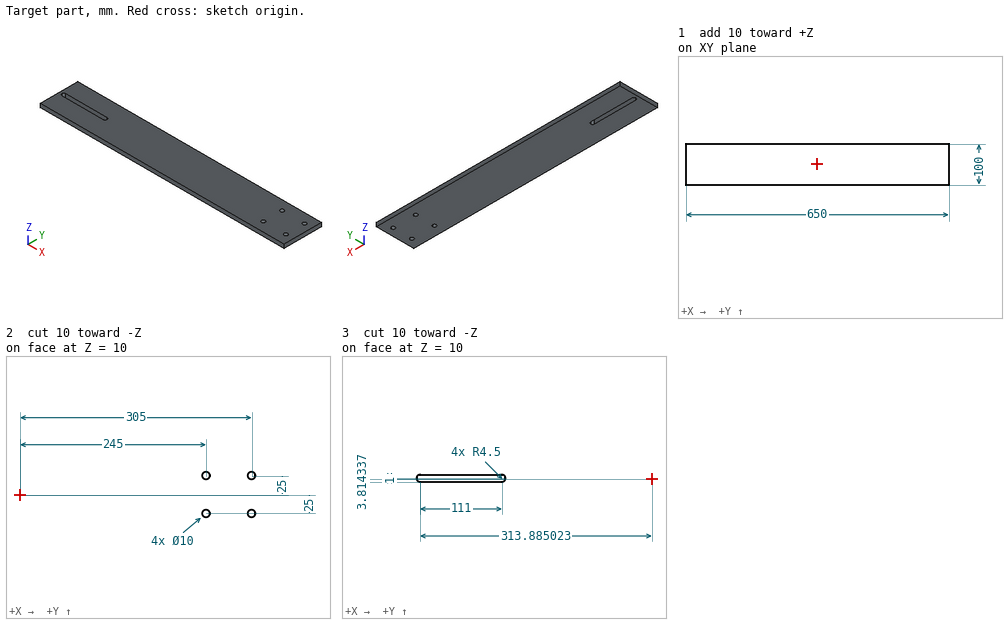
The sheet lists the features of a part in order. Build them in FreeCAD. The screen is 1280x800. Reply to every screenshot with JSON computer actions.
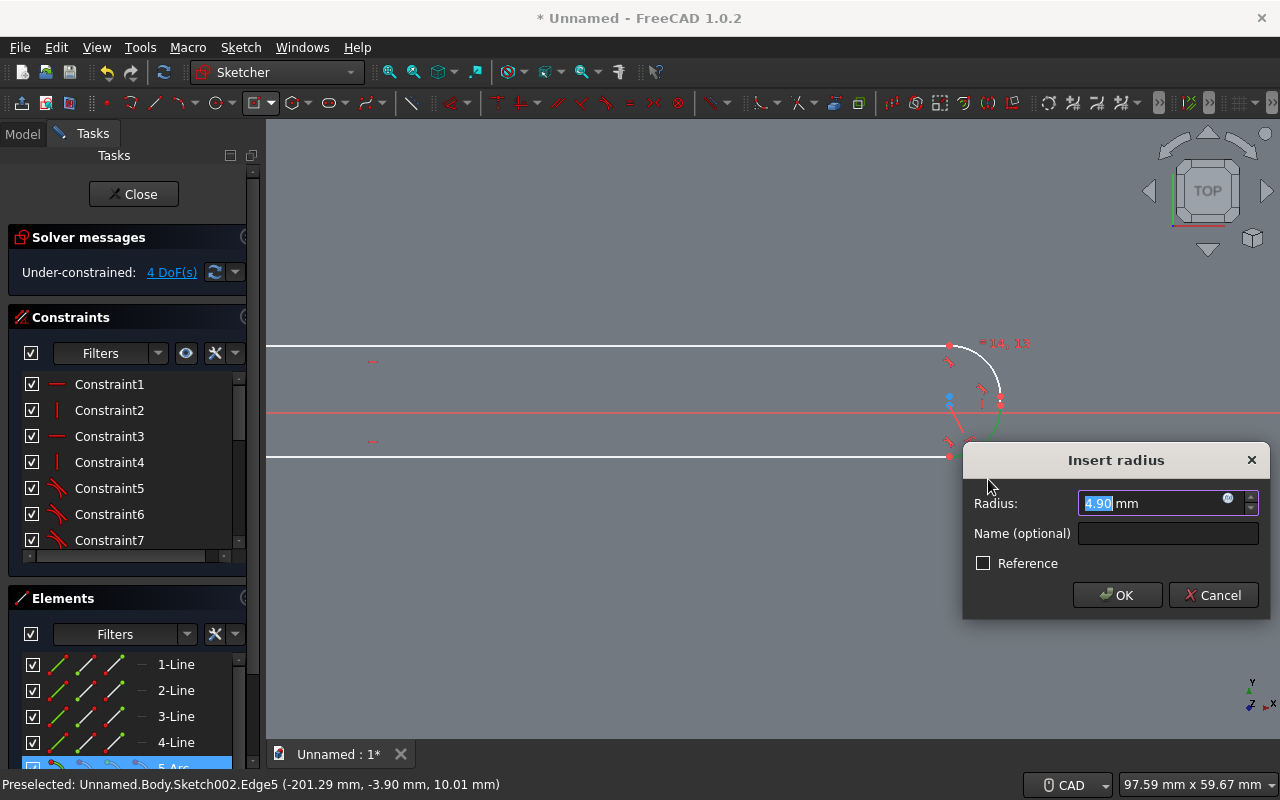
{"action": "type", "text": "4.5"}
{"action": "key", "text": "Return"}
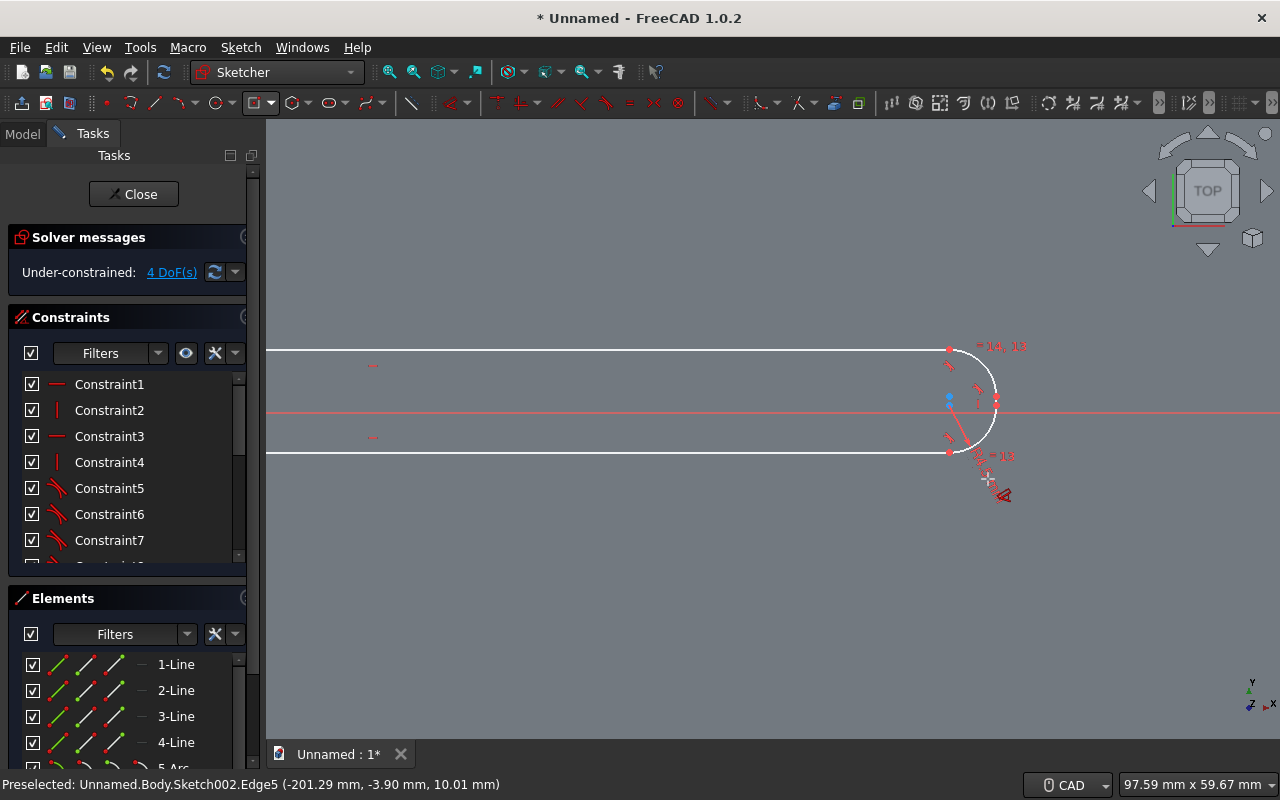
{"action": "scroll", "coordinate": [996, 401], "scroll_direction": "up", "scroll_amount": 7}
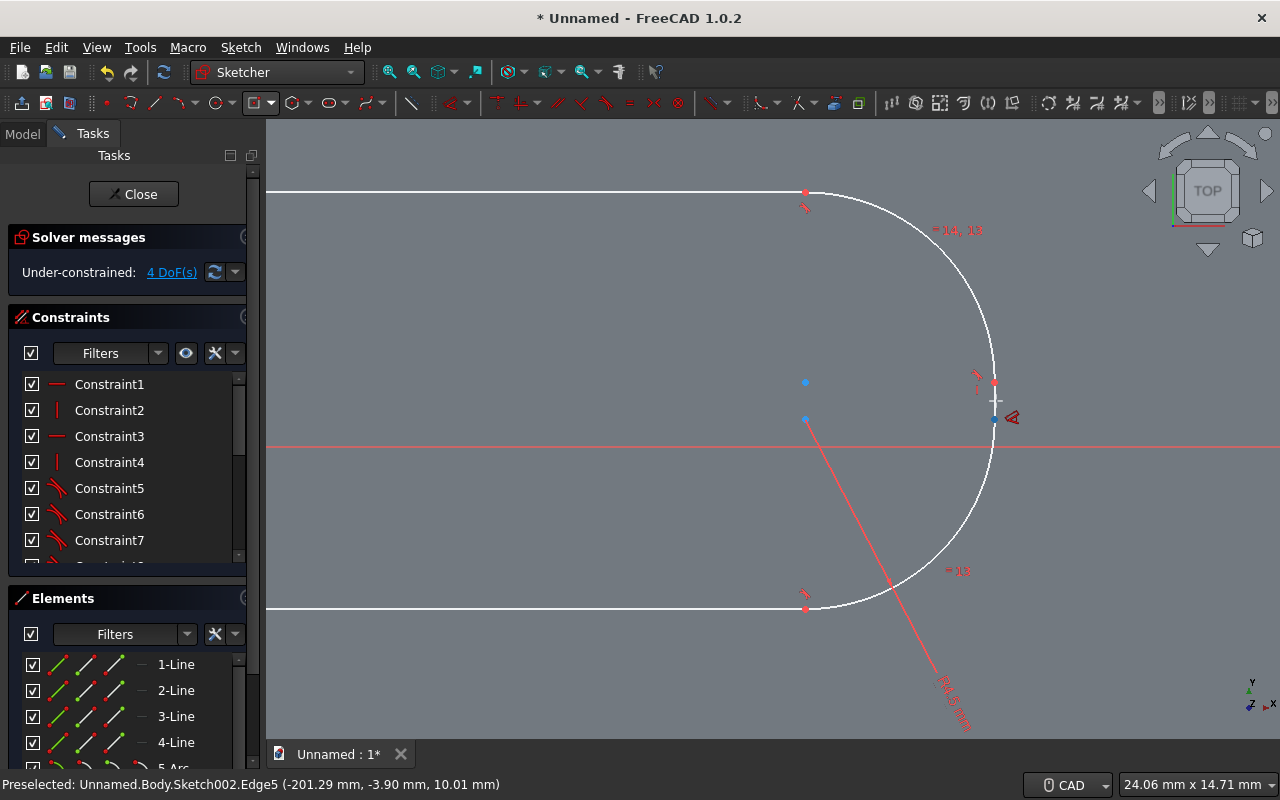
{"action": "left_click", "coordinate": [995, 401]}
{"action": "left_click", "coordinate": [1029, 401]}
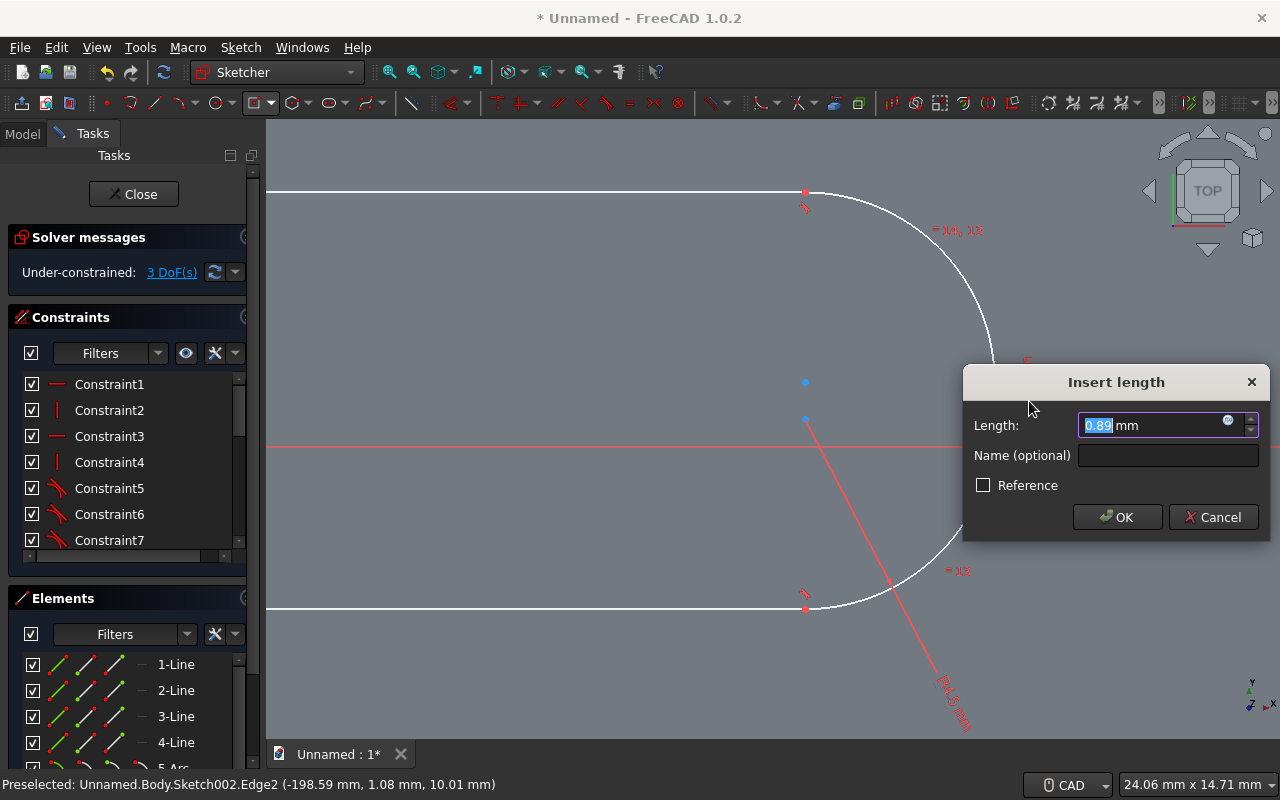
{"action": "type", "text": "1"}
{"action": "key", "text": "Return"}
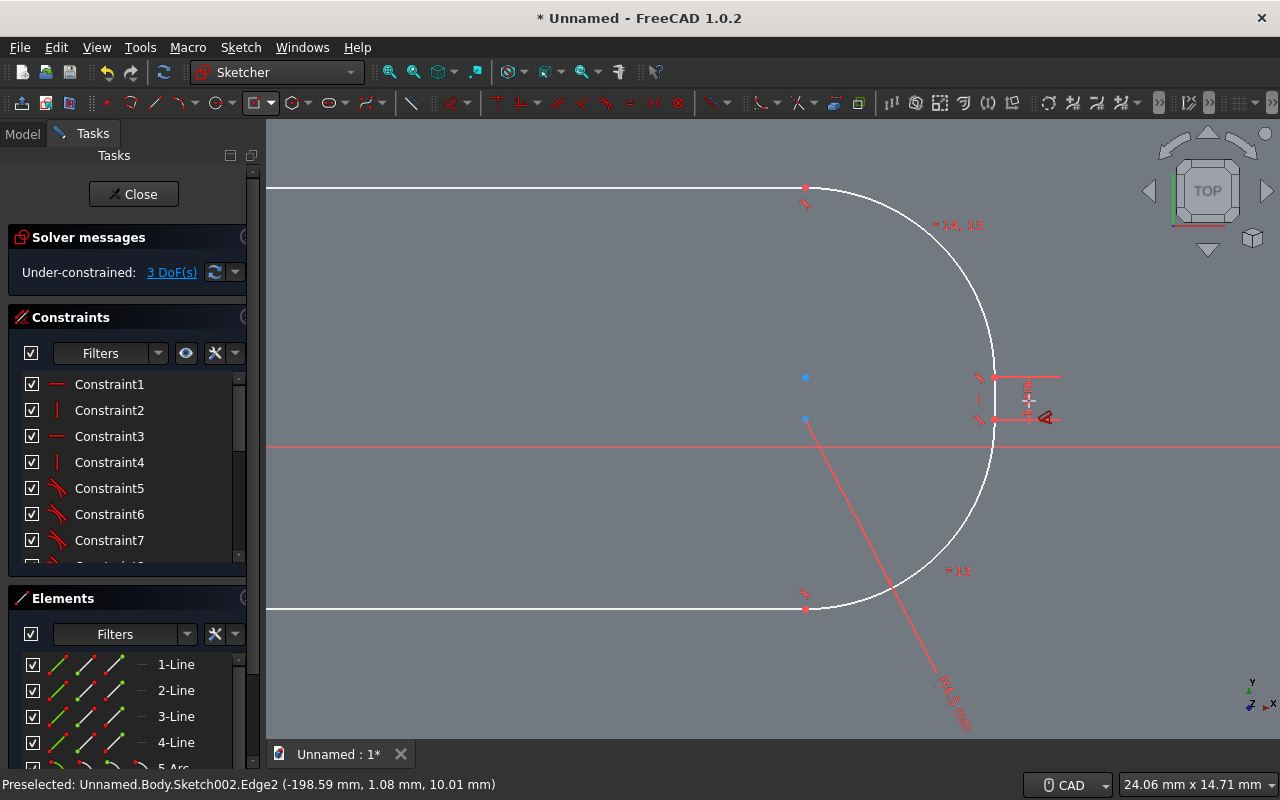
{"action": "scroll", "coordinate": [982, 433], "scroll_direction": "down", "scroll_amount": 11}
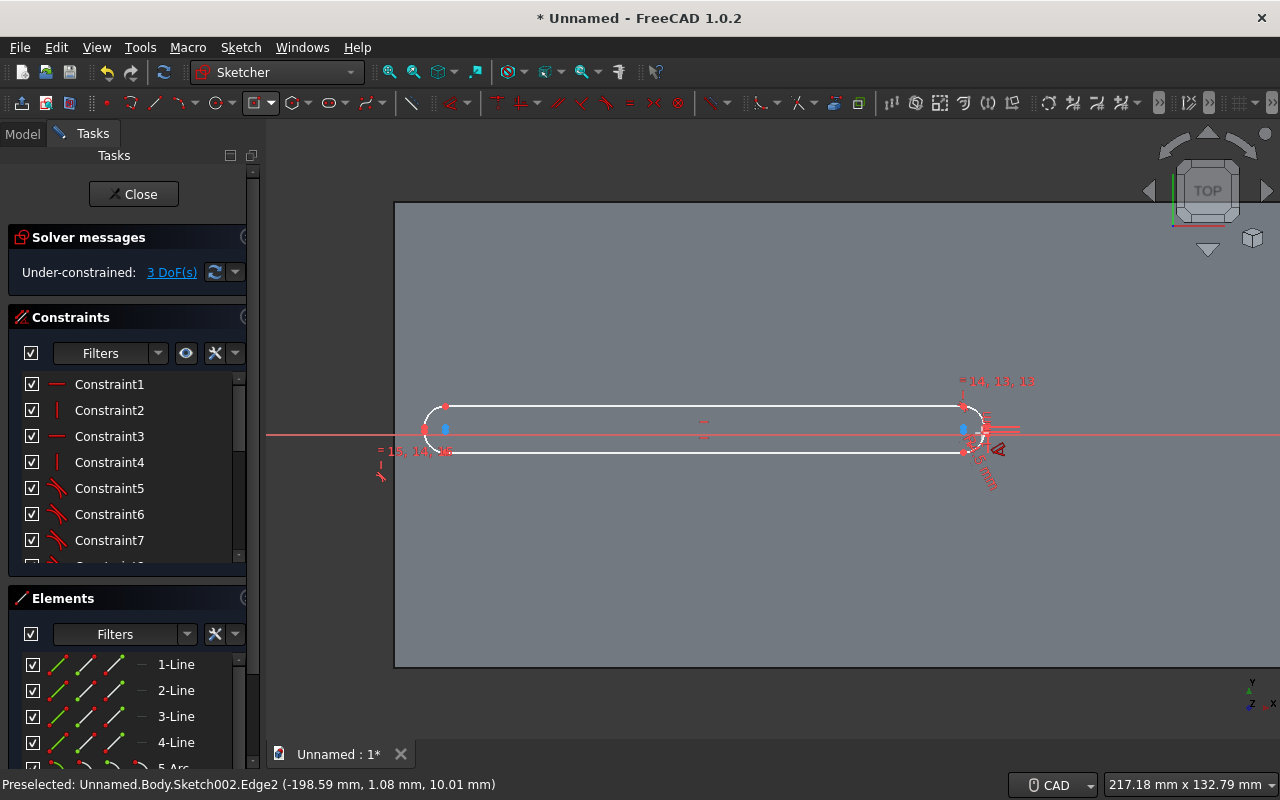
{"action": "left_click", "coordinate": [601, 453]}
{"action": "left_click", "coordinate": [704, 487]}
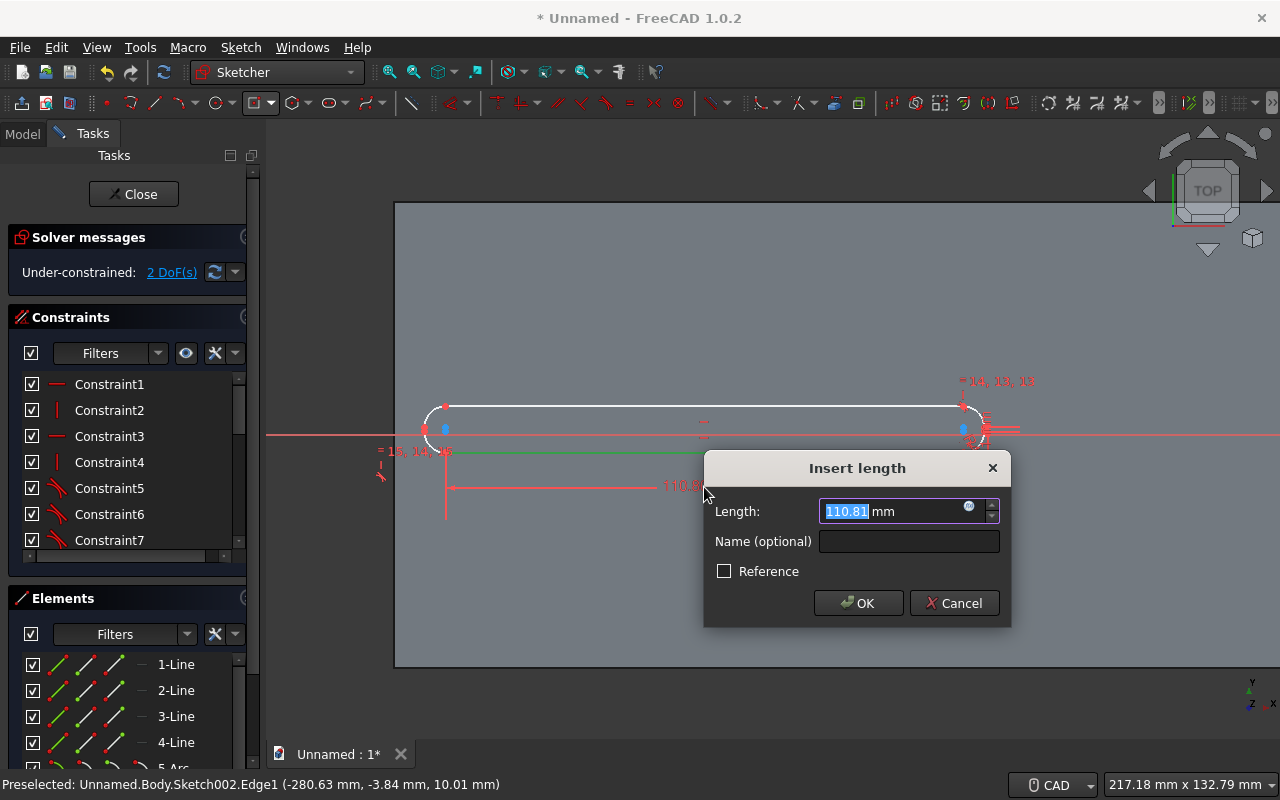
{"action": "type", "text": "111"}
{"action": "key", "text": "Return"}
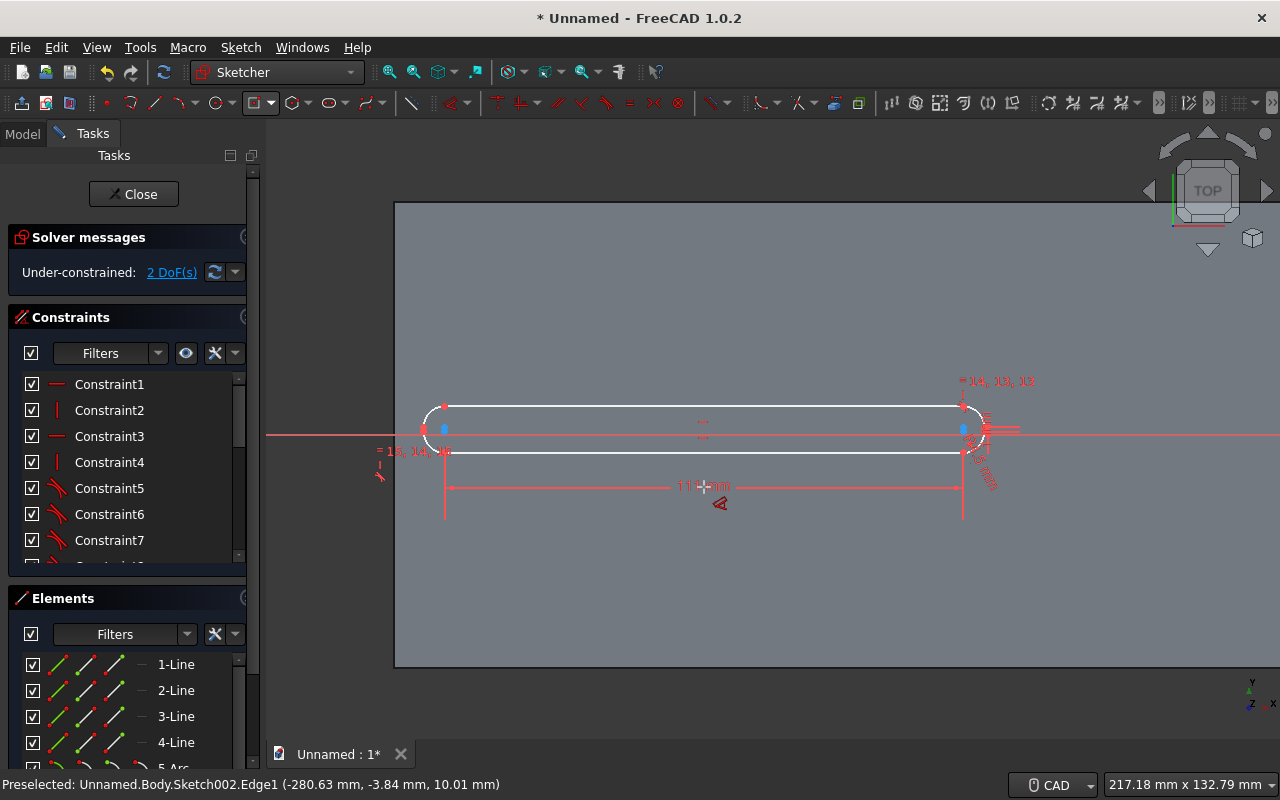
{"action": "scroll", "coordinate": [445, 453], "scroll_direction": "up", "scroll_amount": 5}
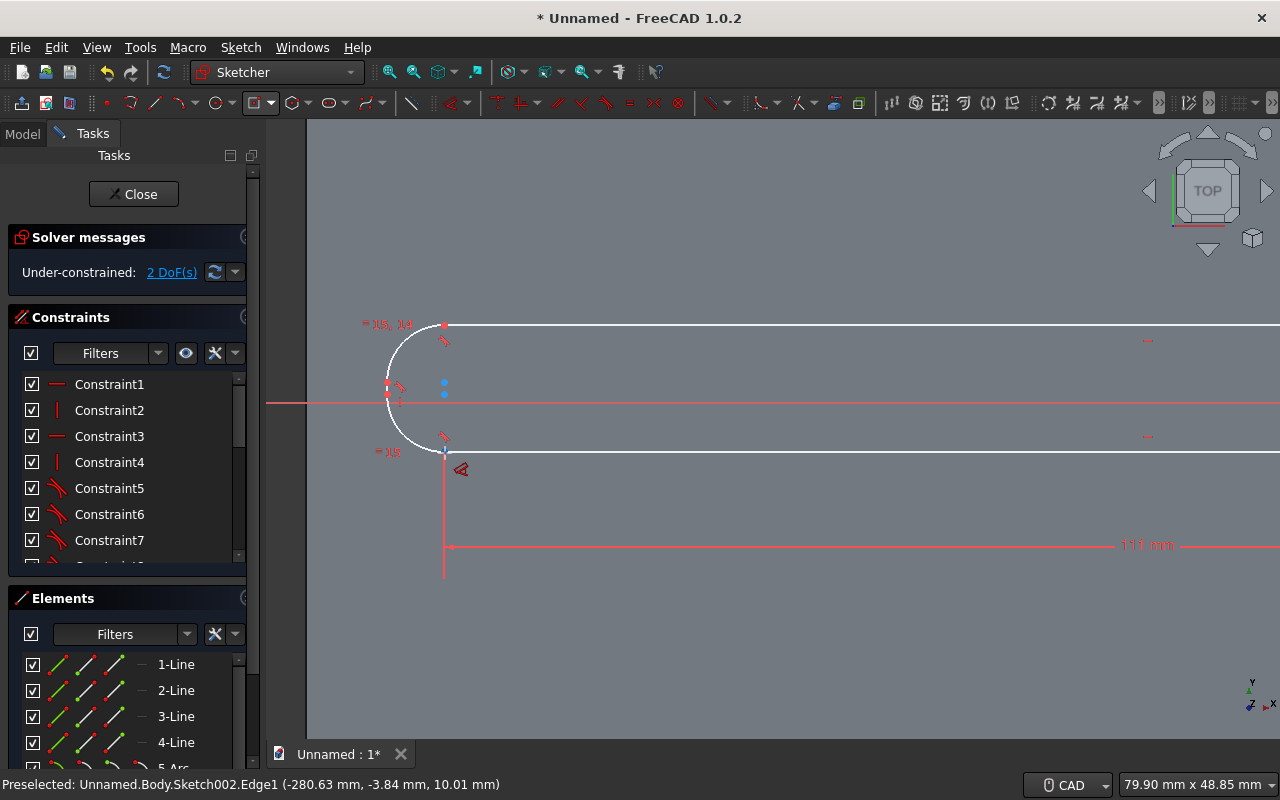
{"action": "left_click", "coordinate": [444, 452]}
{"action": "left_click", "coordinate": [410, 416]}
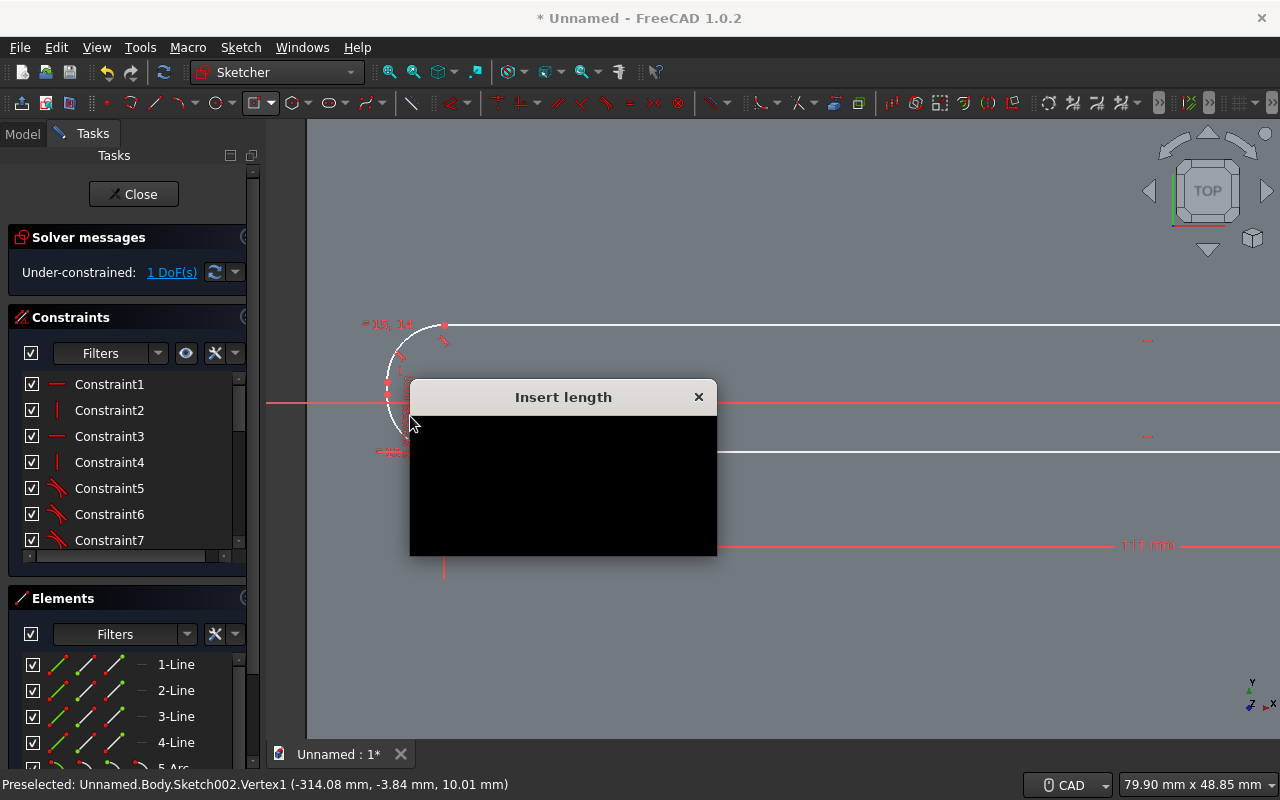
{"action": "type", "text": "3.814337"}
{"action": "key", "text": "Return"}